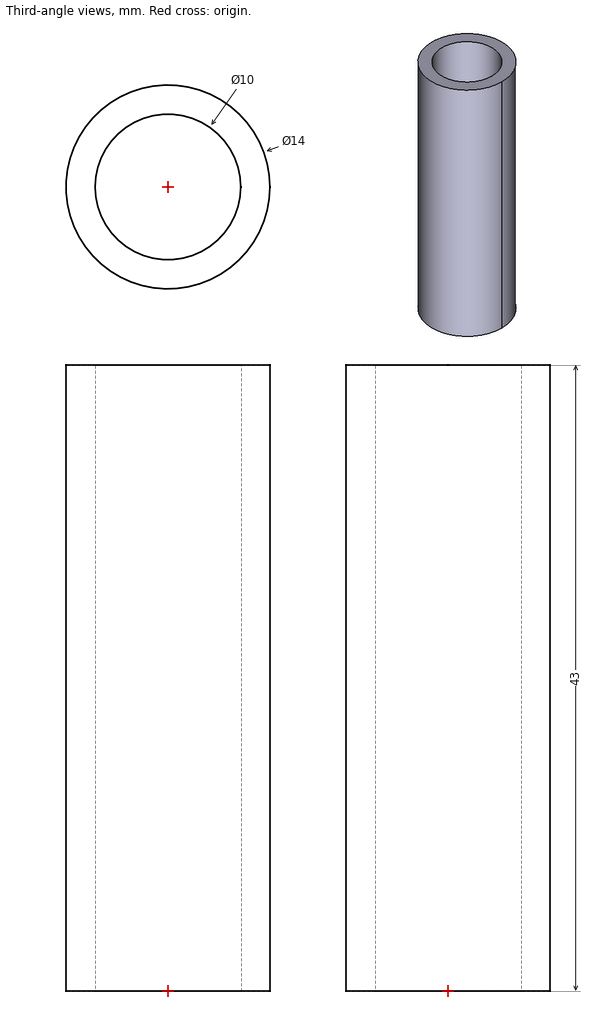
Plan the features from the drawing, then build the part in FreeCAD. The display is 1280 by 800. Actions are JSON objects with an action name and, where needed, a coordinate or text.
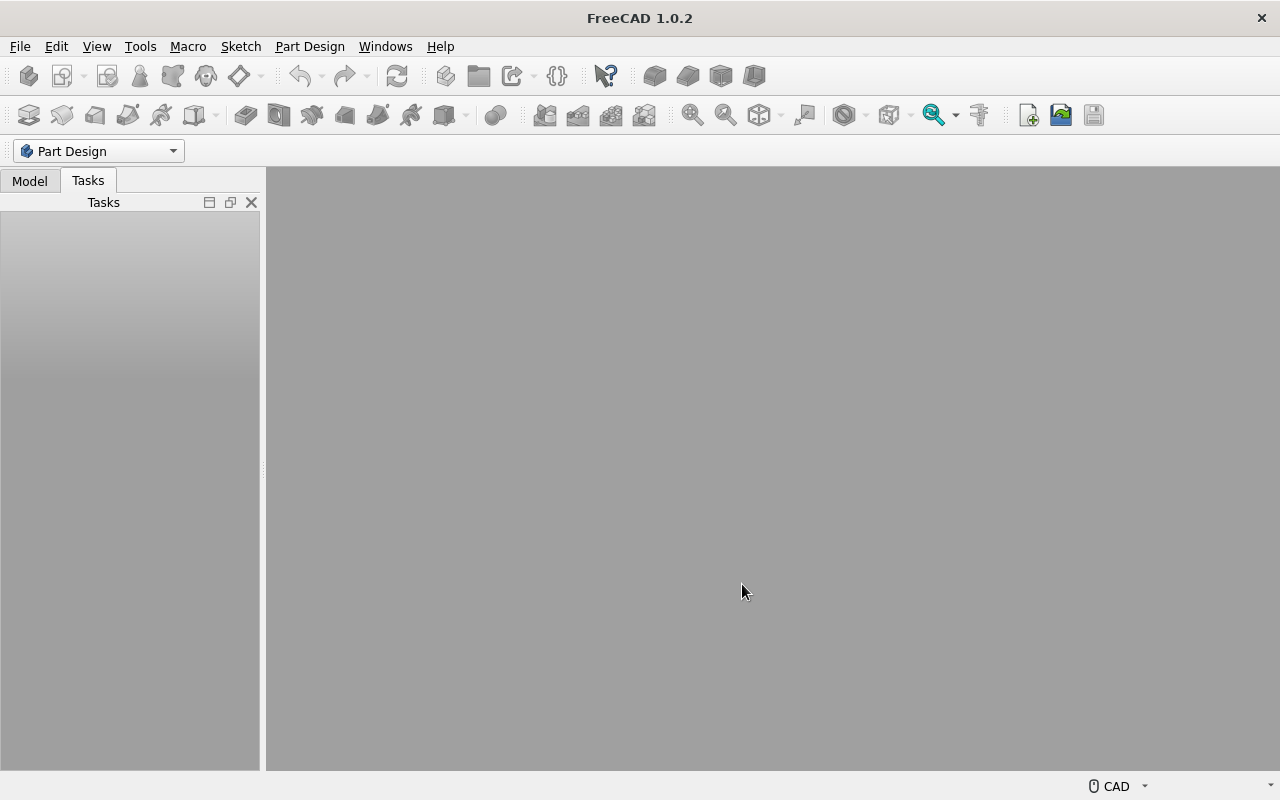
{"action": "left_click", "coordinate": [1028, 116]}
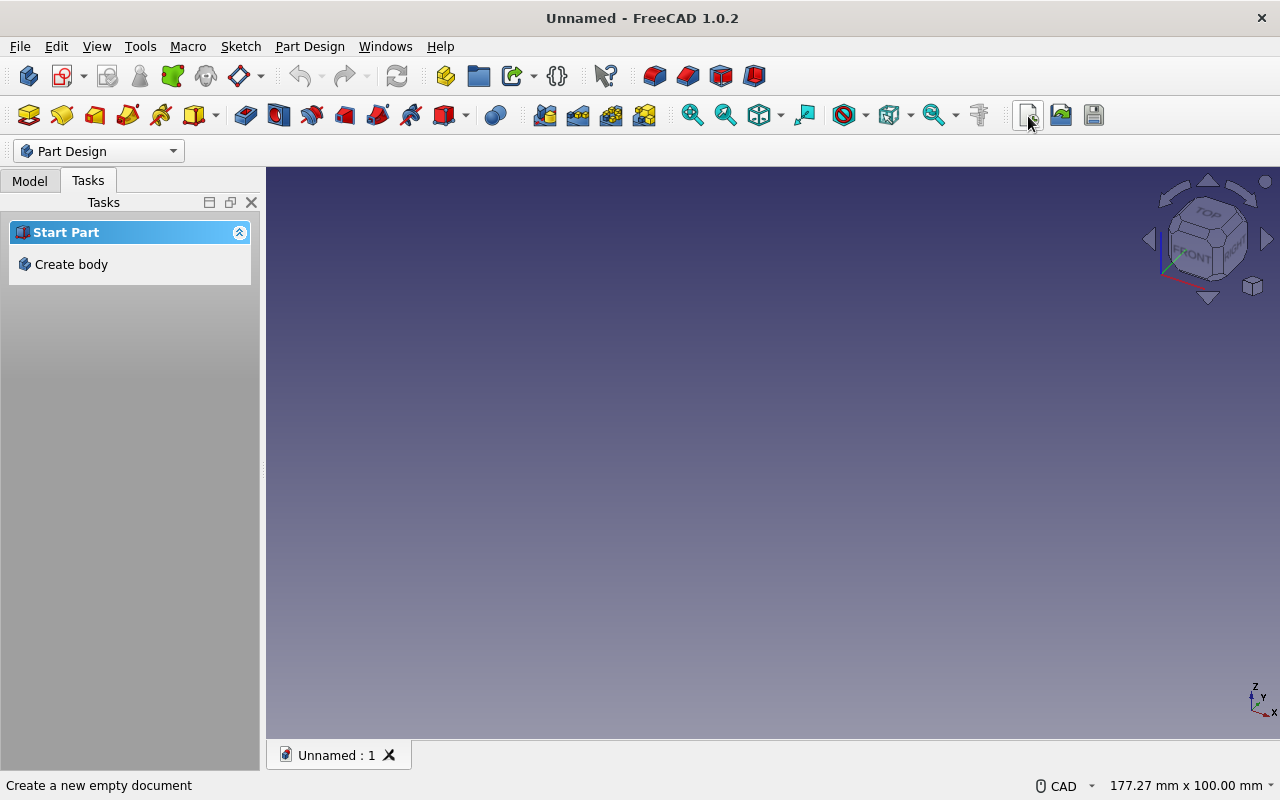
{"action": "left_click", "coordinate": [62, 76]}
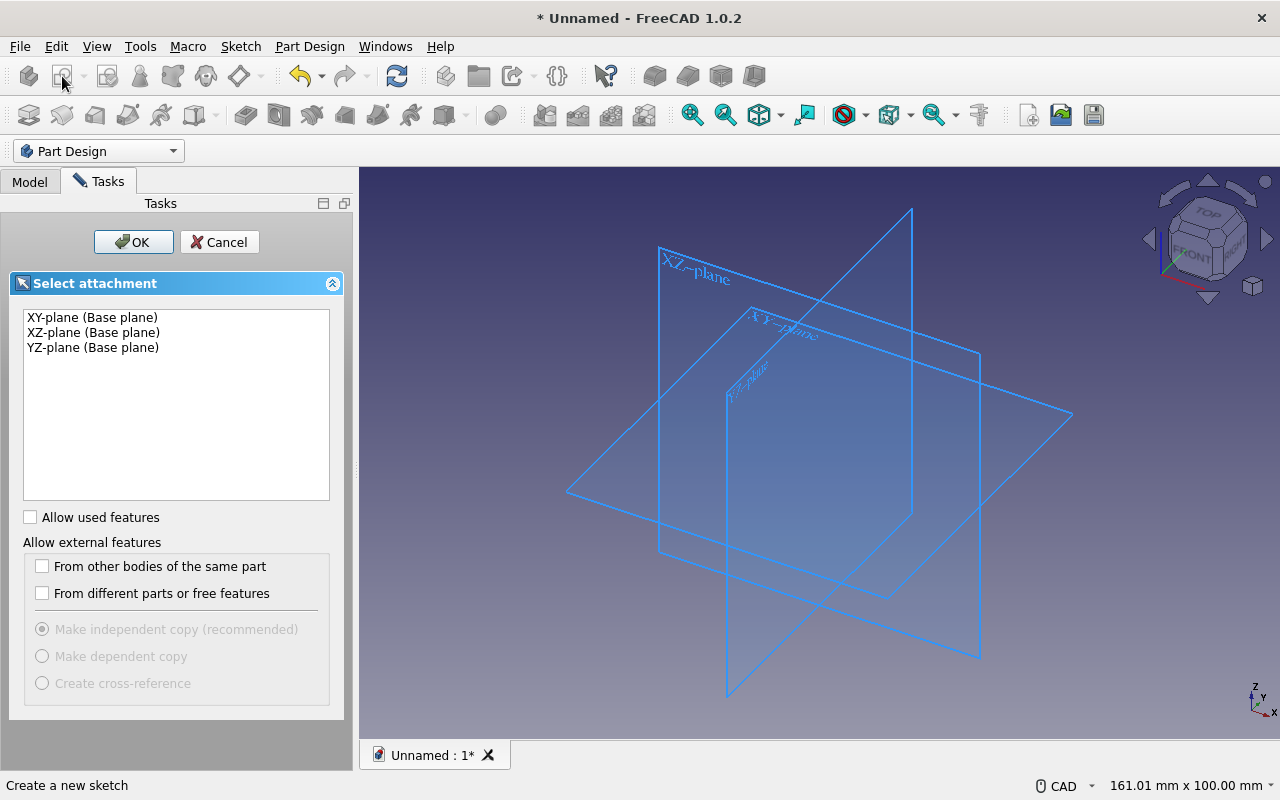
{"action": "left_click", "coordinate": [84, 318]}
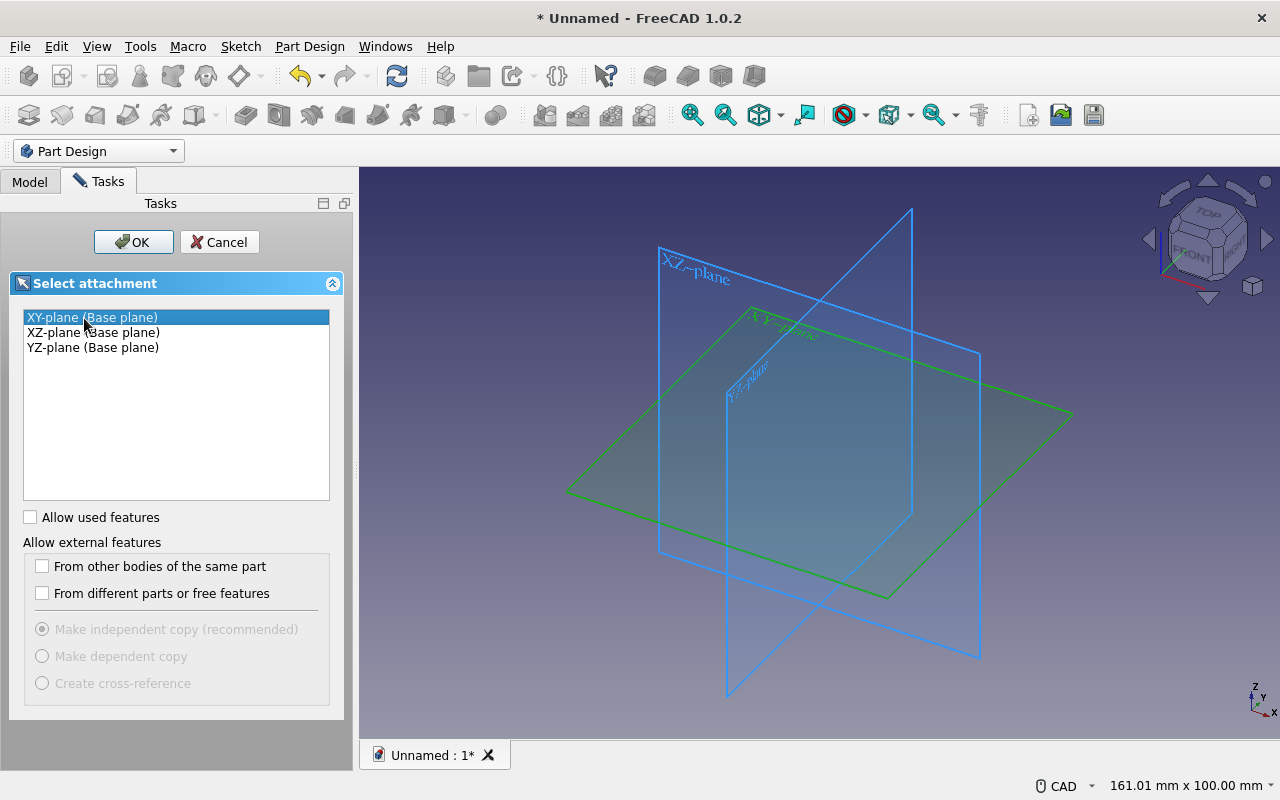
{"action": "left_click", "coordinate": [134, 242]}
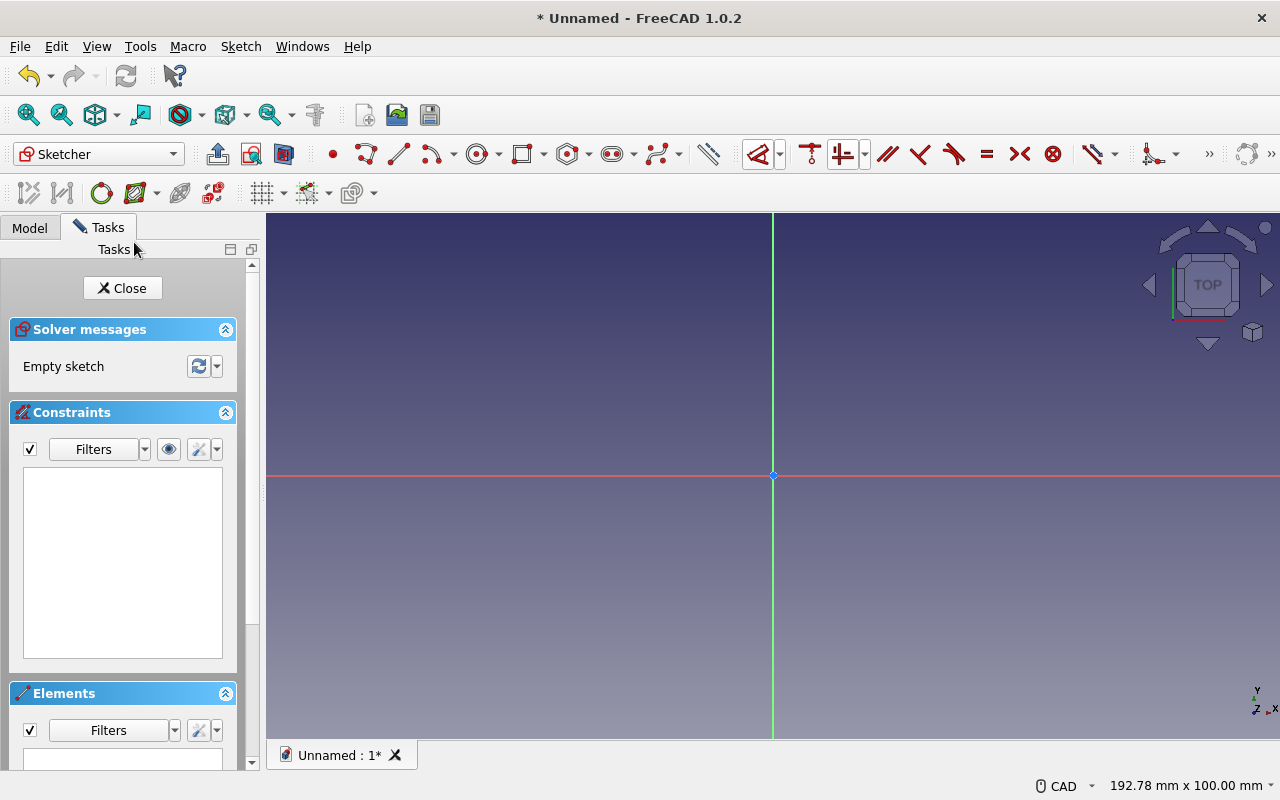
{"action": "scroll", "coordinate": [790, 476], "scroll_direction": "up", "scroll_amount": 8}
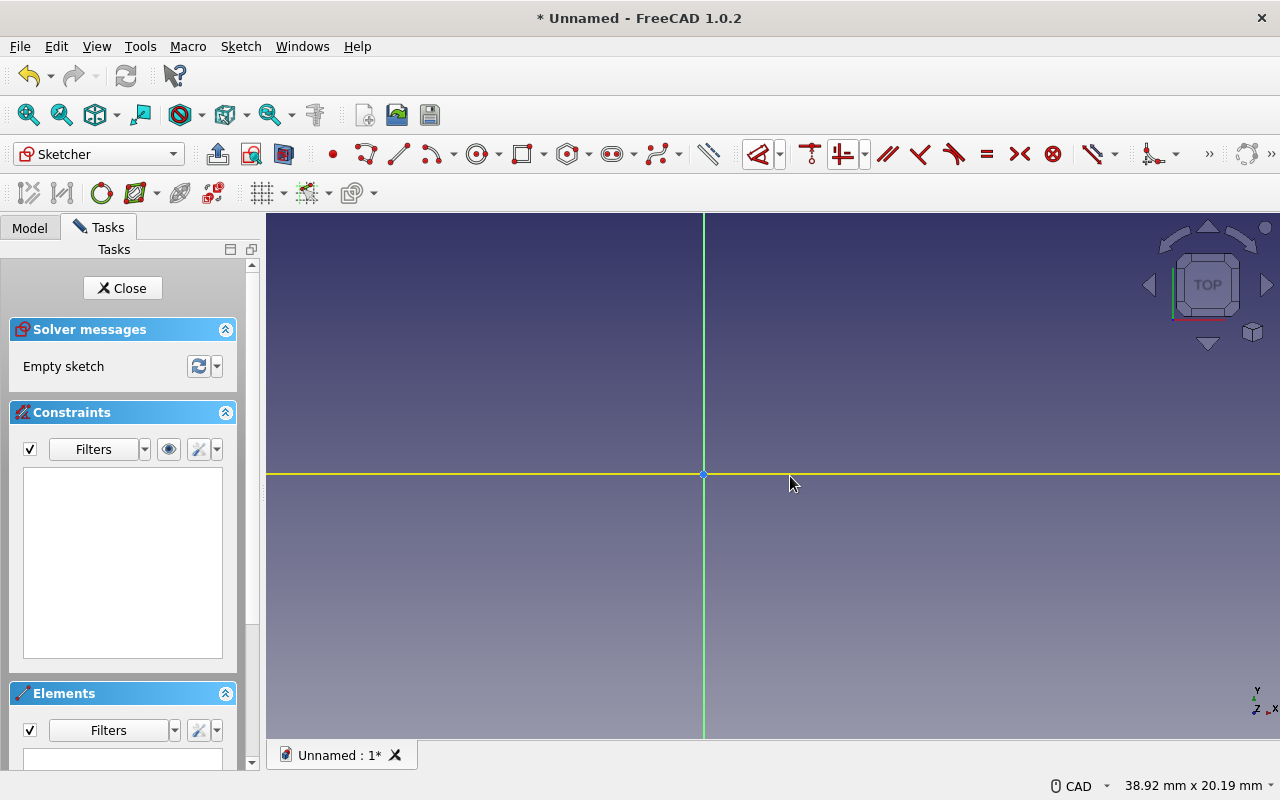
{"action": "left_click", "coordinate": [476, 154]}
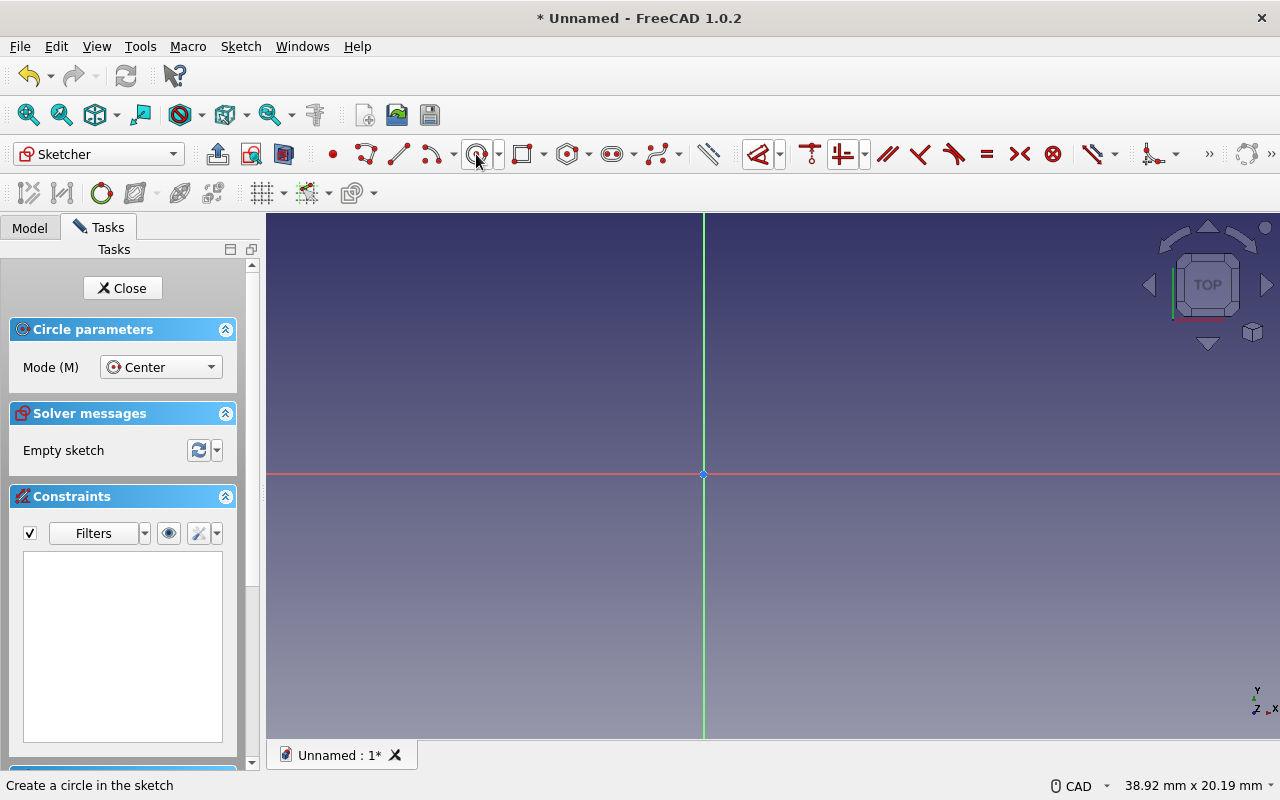
{"action": "left_click", "coordinate": [704, 474]}
{"action": "left_click", "coordinate": [833, 345]}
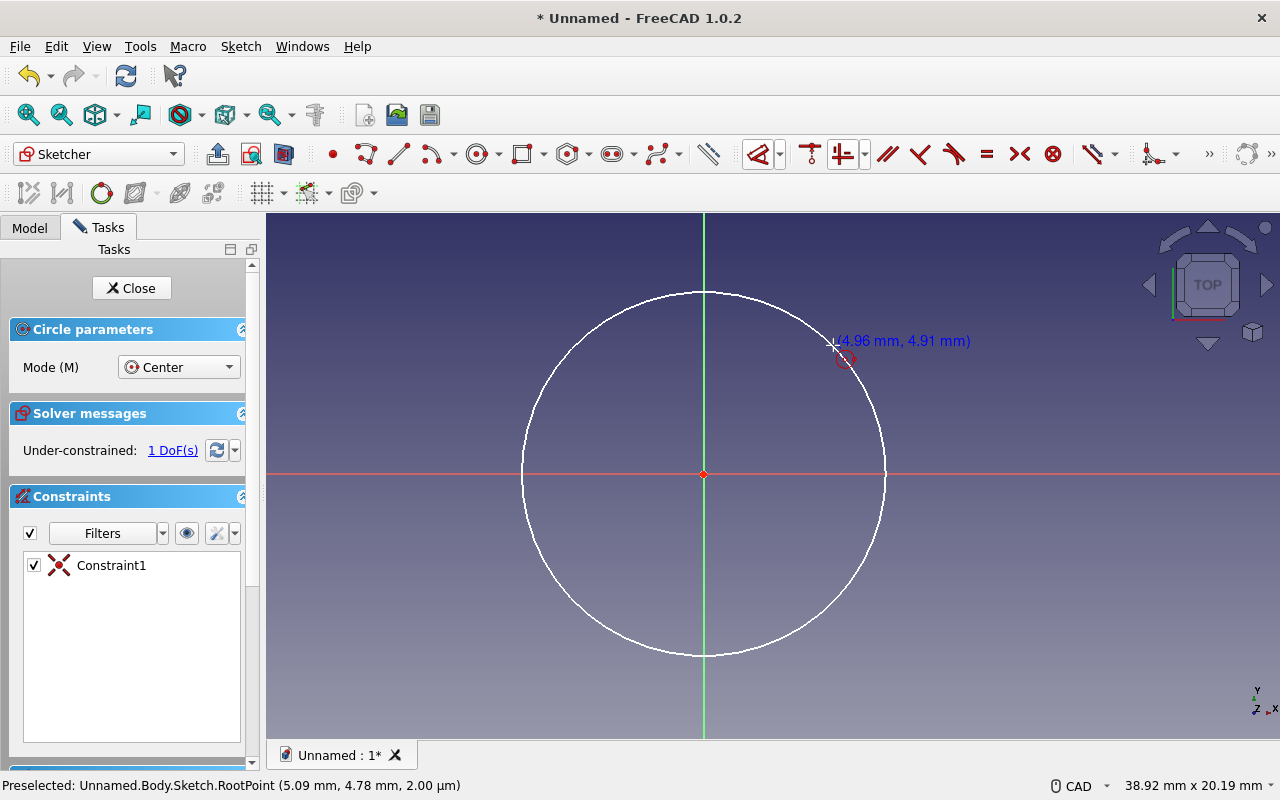
{"action": "left_click", "coordinate": [704, 474]}
{"action": "left_click", "coordinate": [796, 382]}
{"action": "key", "text": "Escape"}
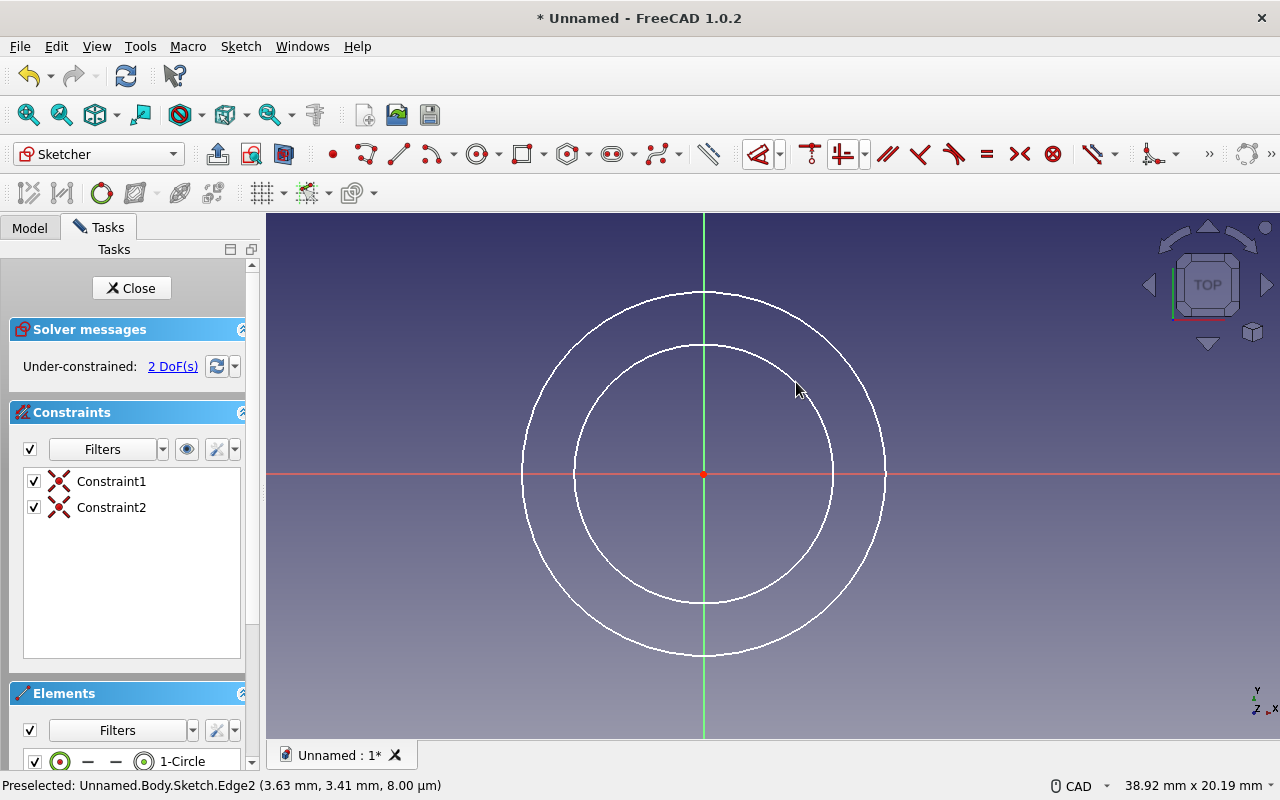
{"action": "left_click", "coordinate": [832, 345]}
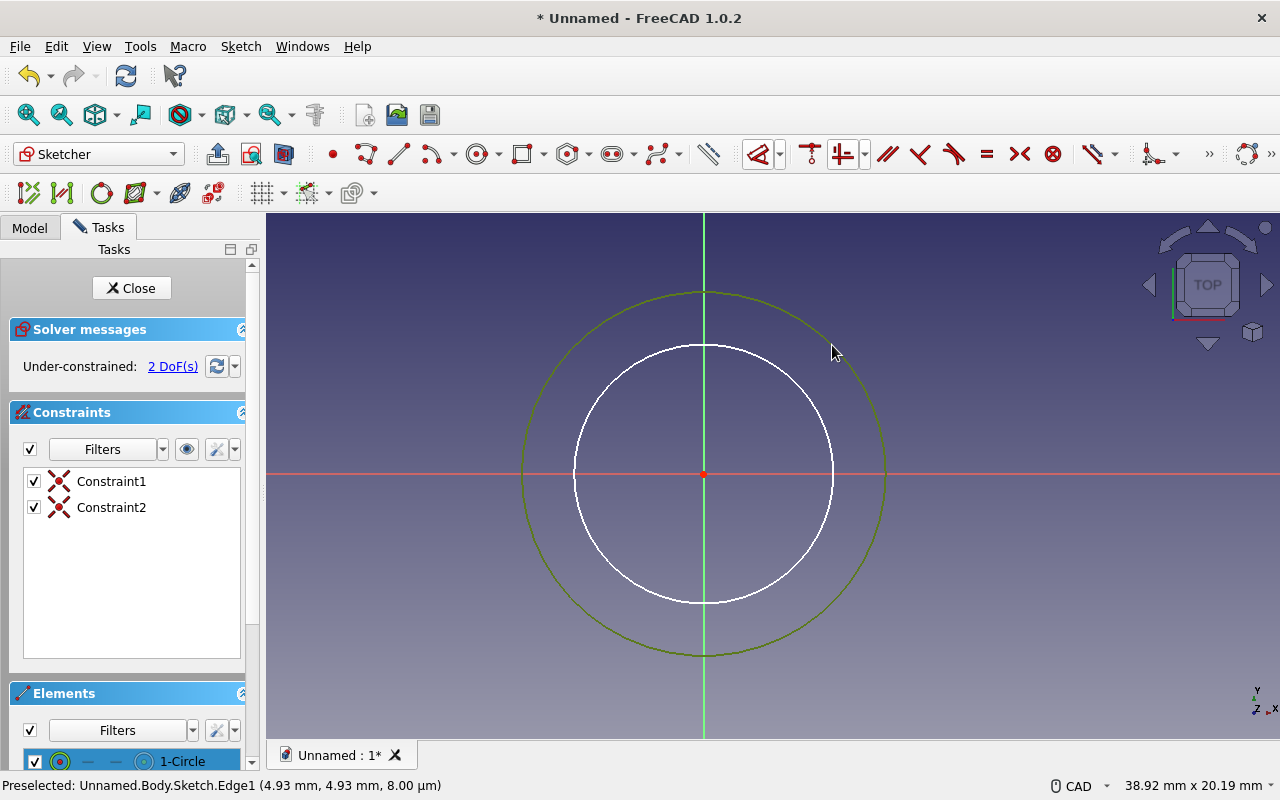
{"action": "left_click", "coordinate": [780, 154]}